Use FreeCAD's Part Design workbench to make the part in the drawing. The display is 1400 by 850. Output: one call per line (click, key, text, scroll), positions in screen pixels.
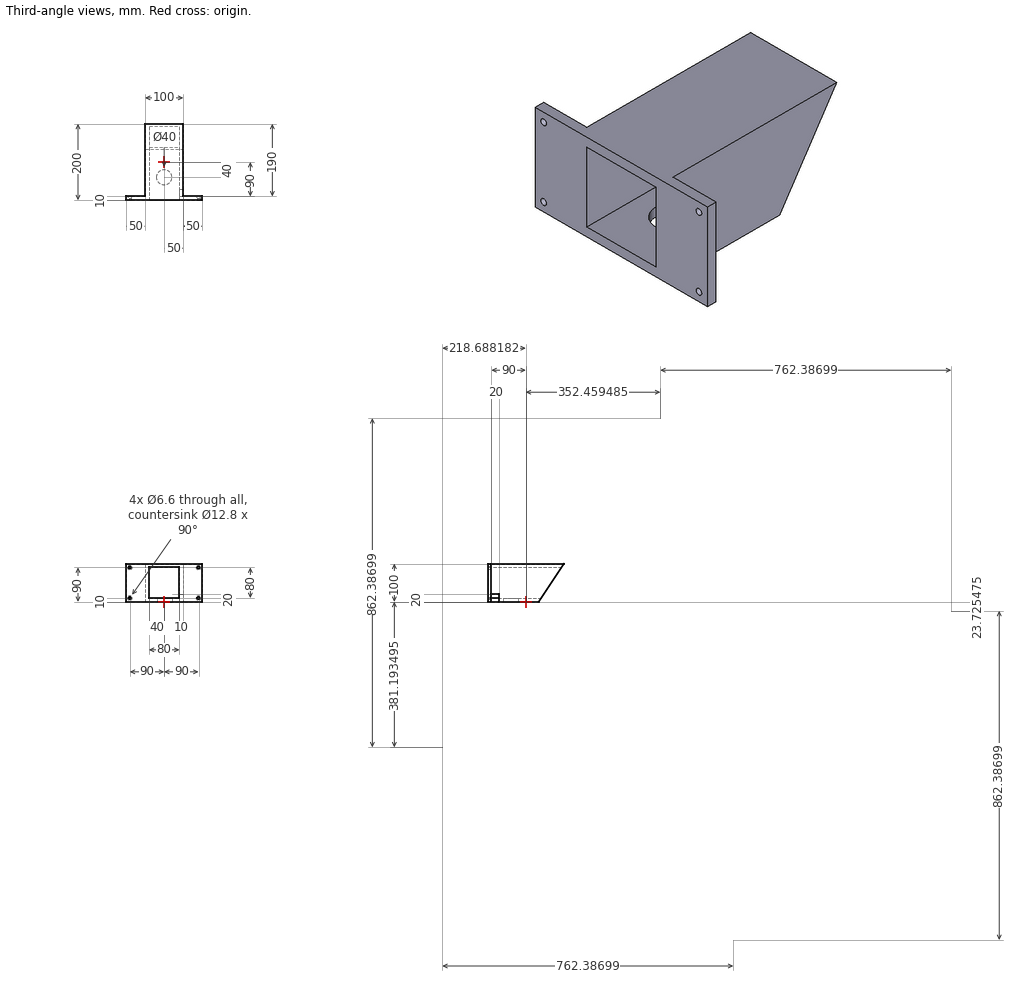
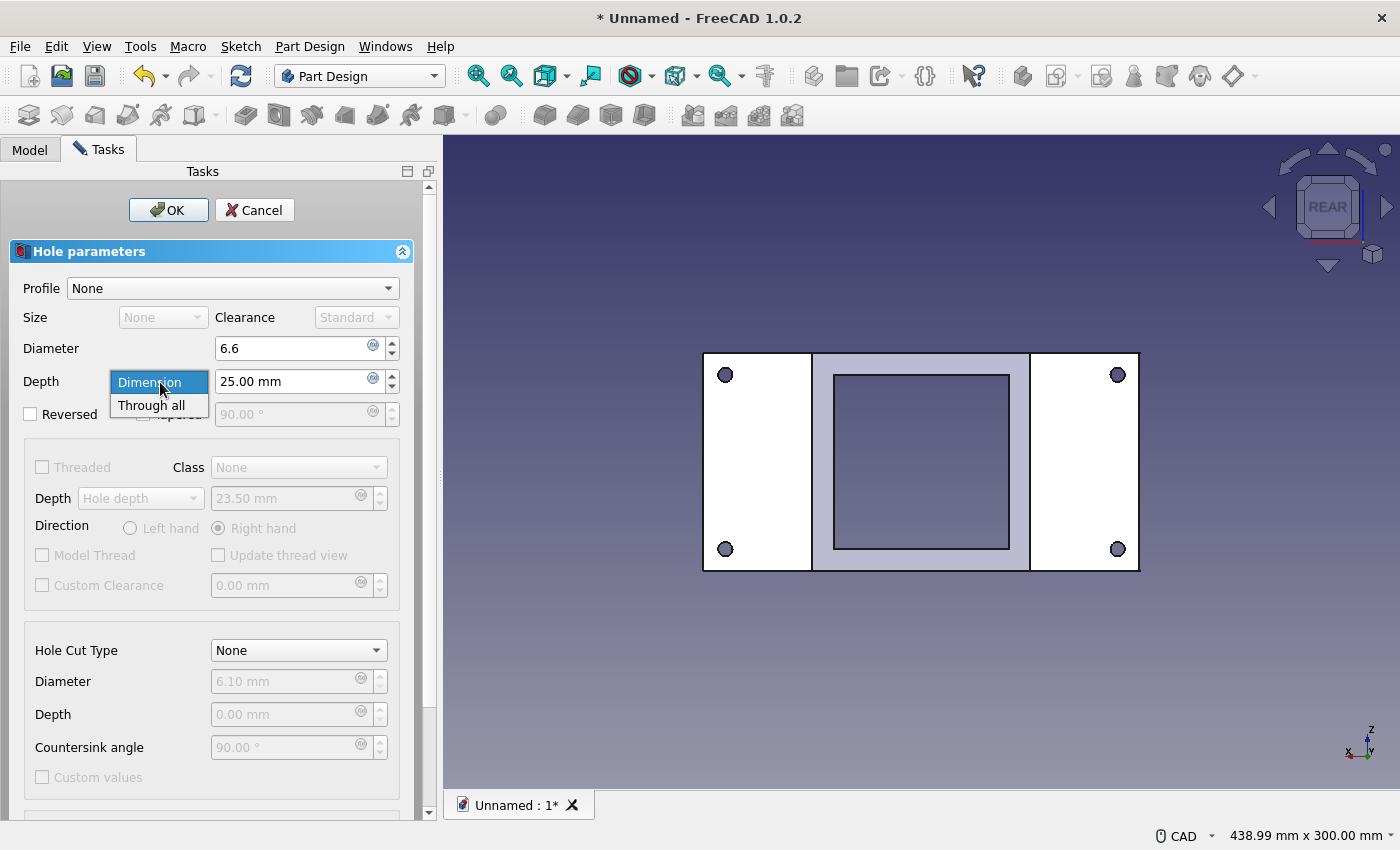
click(158, 406)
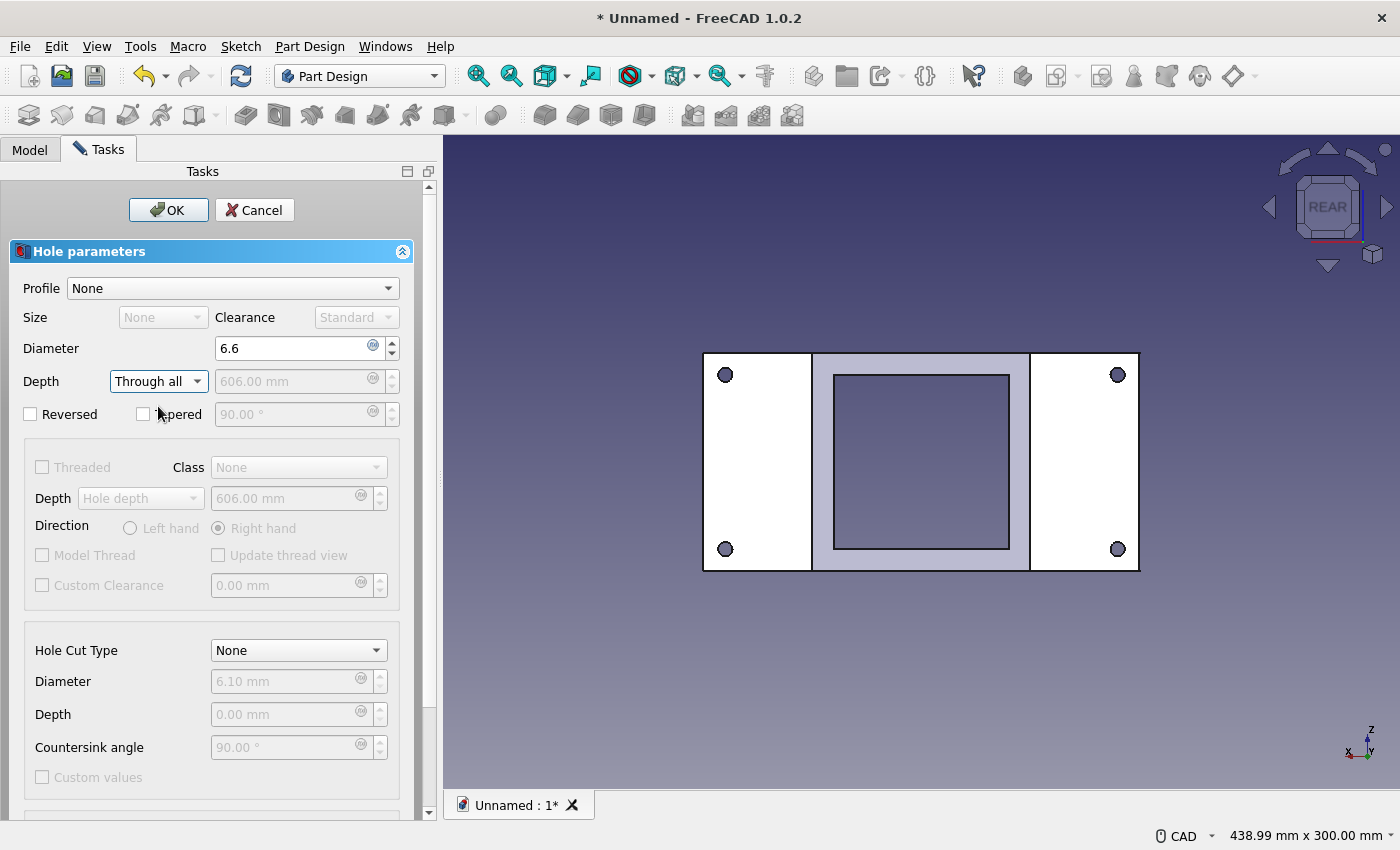
click(300, 650)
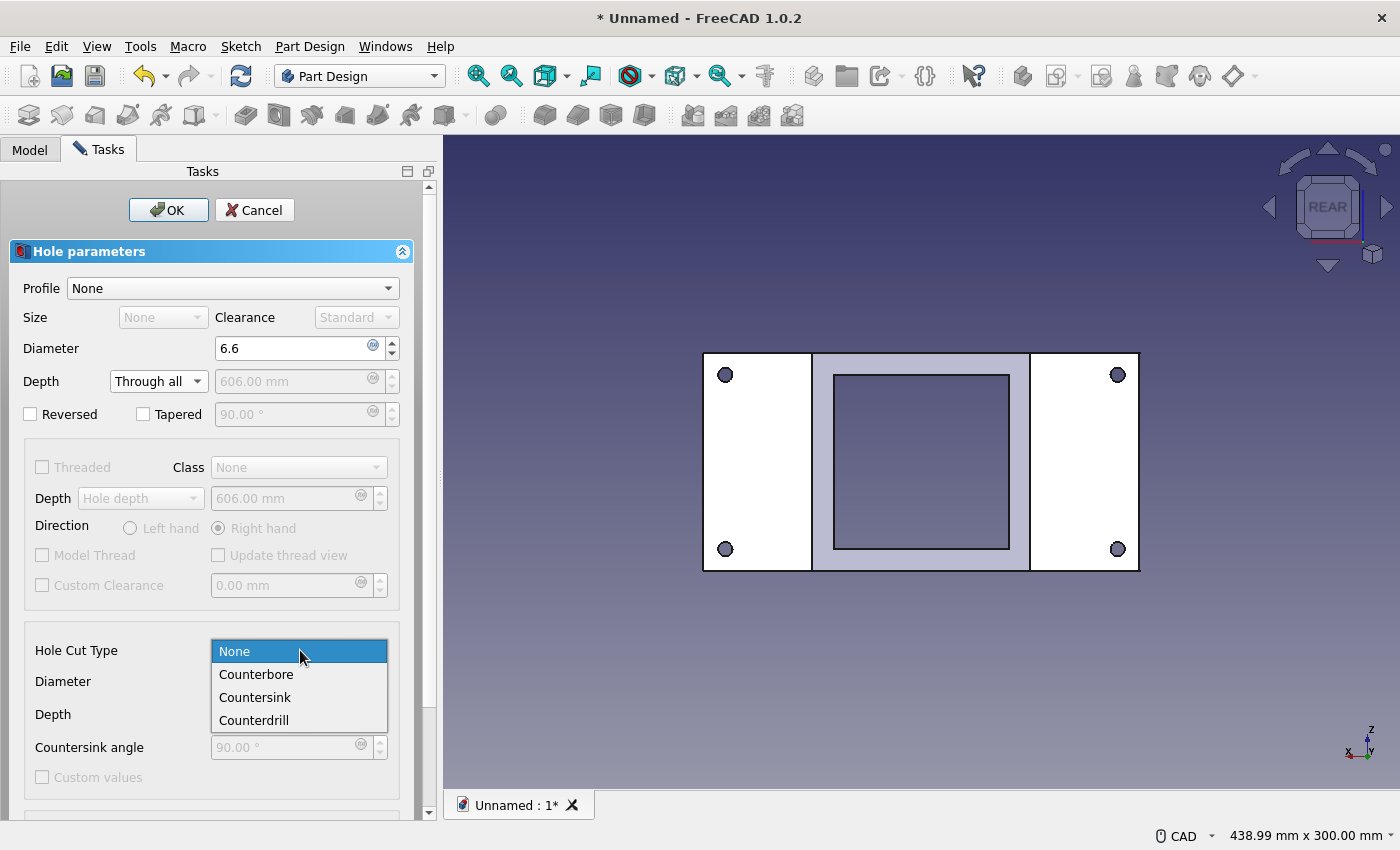
click(298, 698)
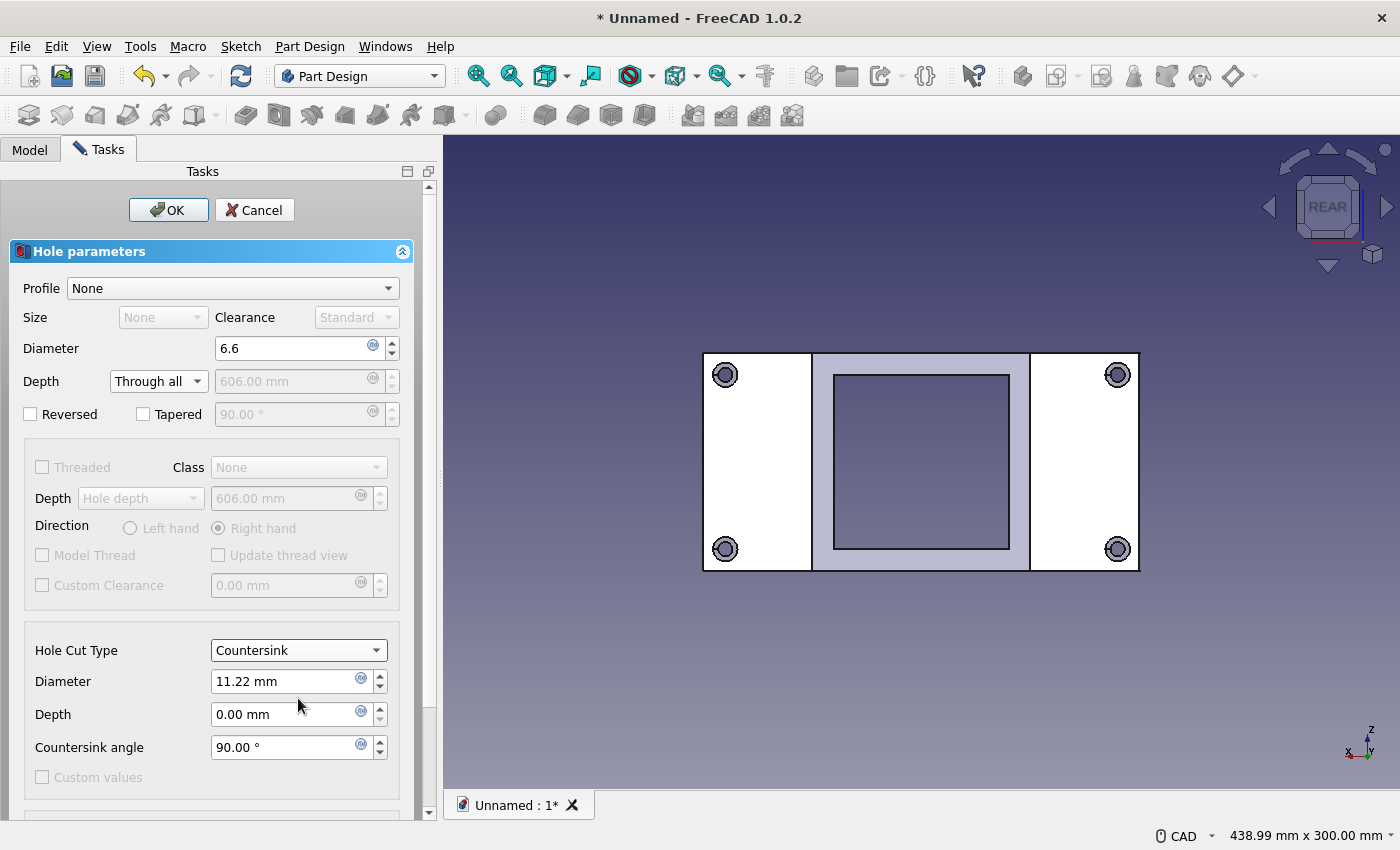
triple_click(292, 682)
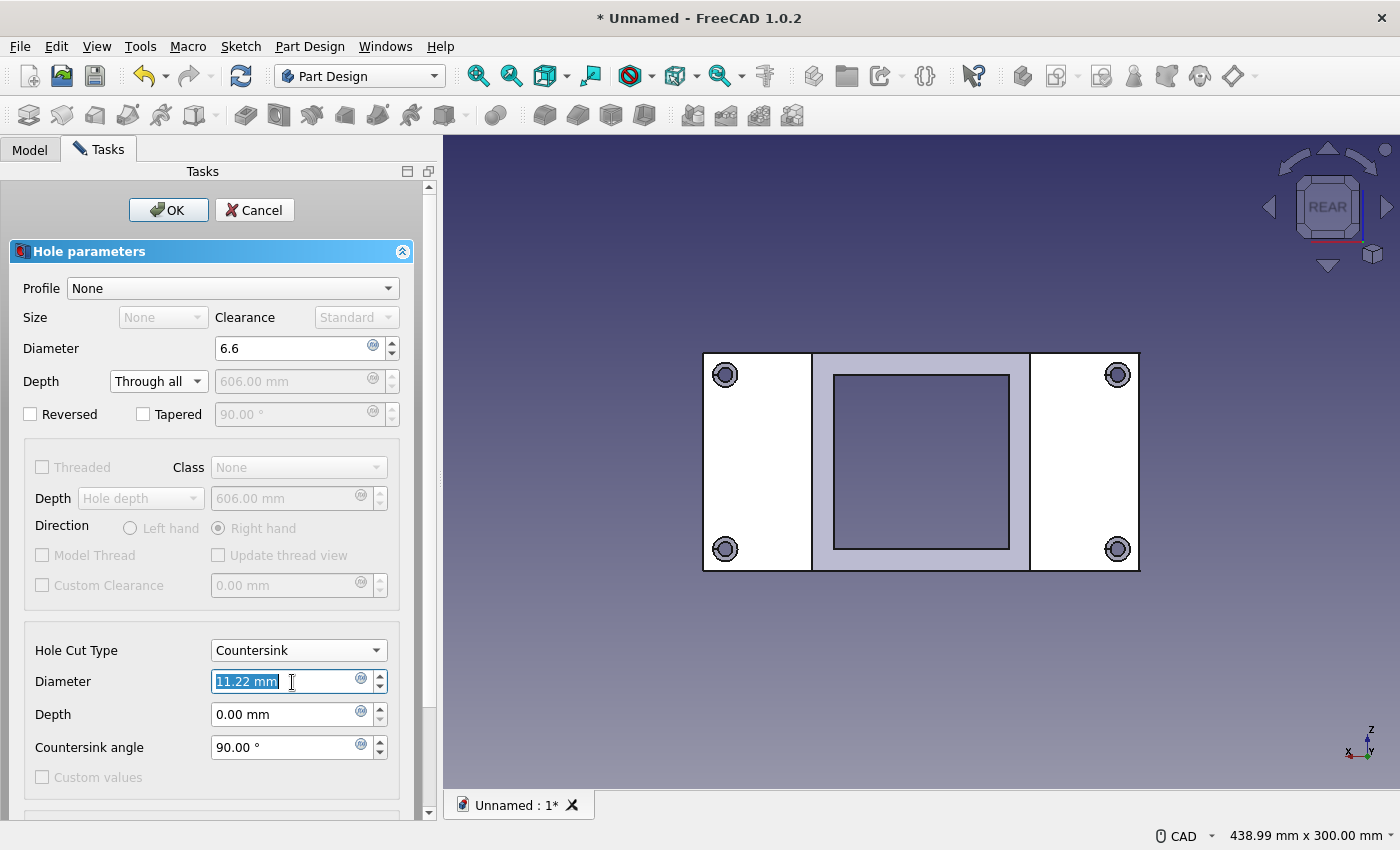
text(12.8)
key(Tab)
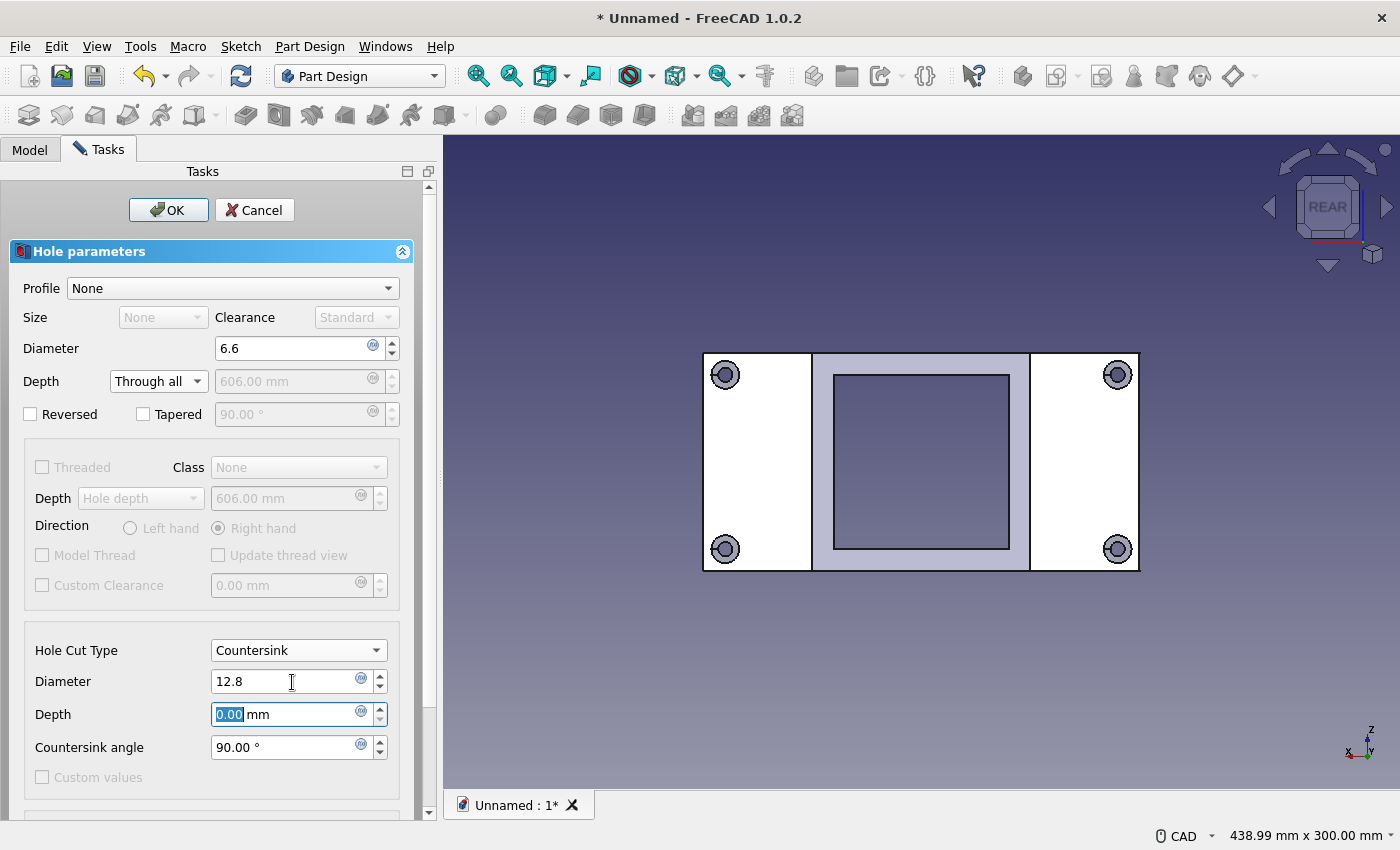
click(169, 210)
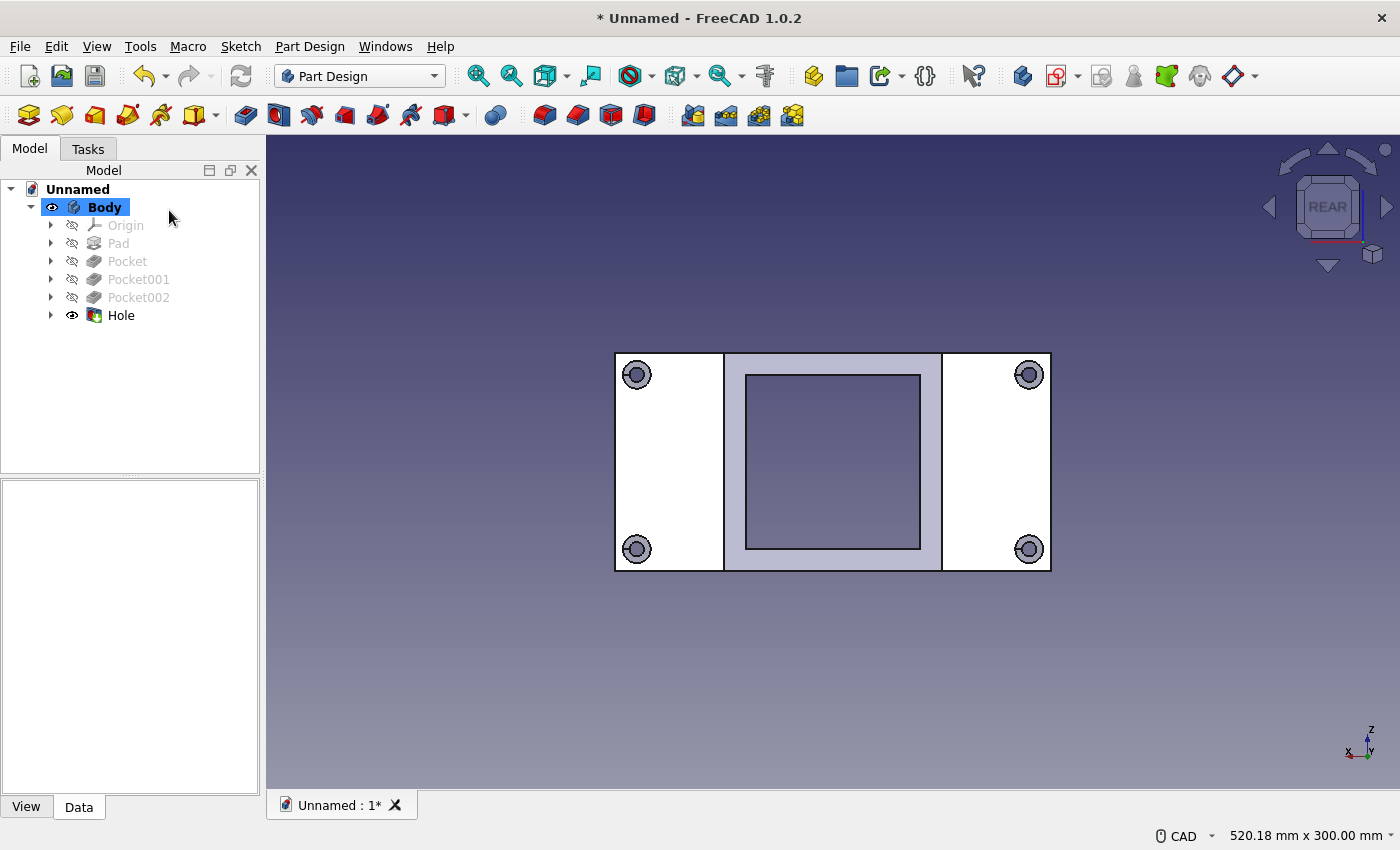
key(v)
key(f)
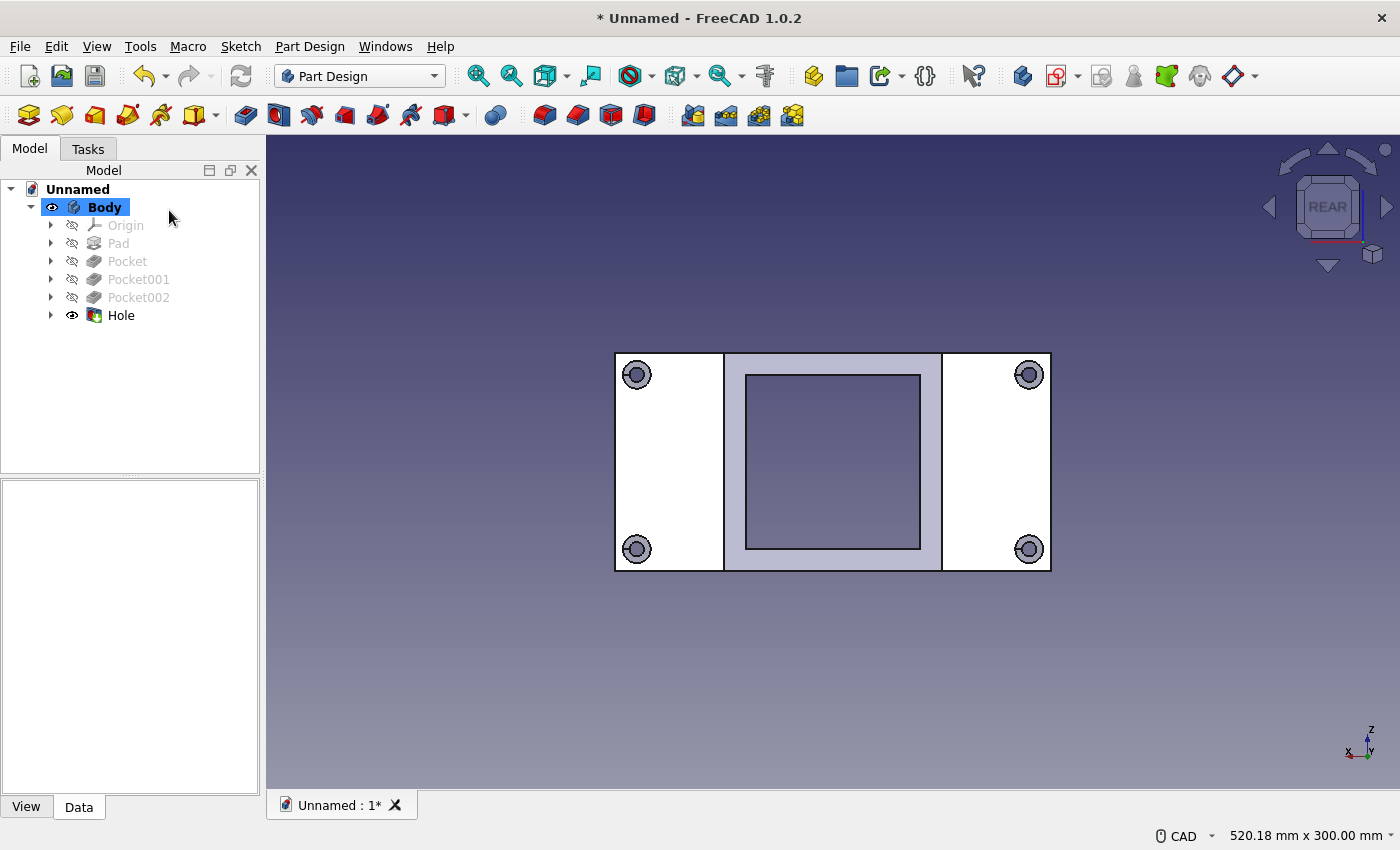
key(0)